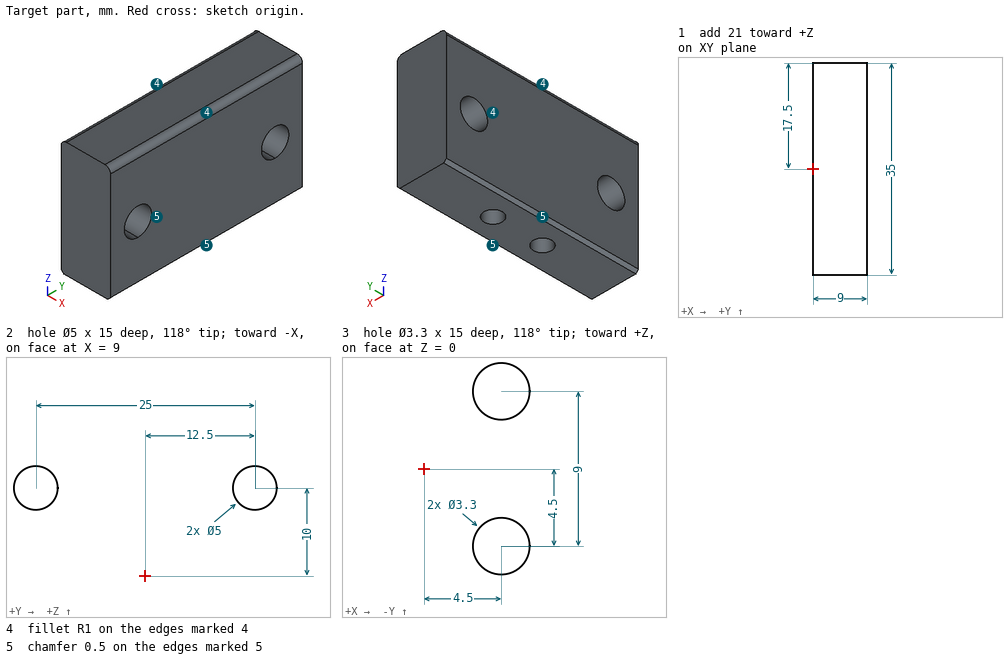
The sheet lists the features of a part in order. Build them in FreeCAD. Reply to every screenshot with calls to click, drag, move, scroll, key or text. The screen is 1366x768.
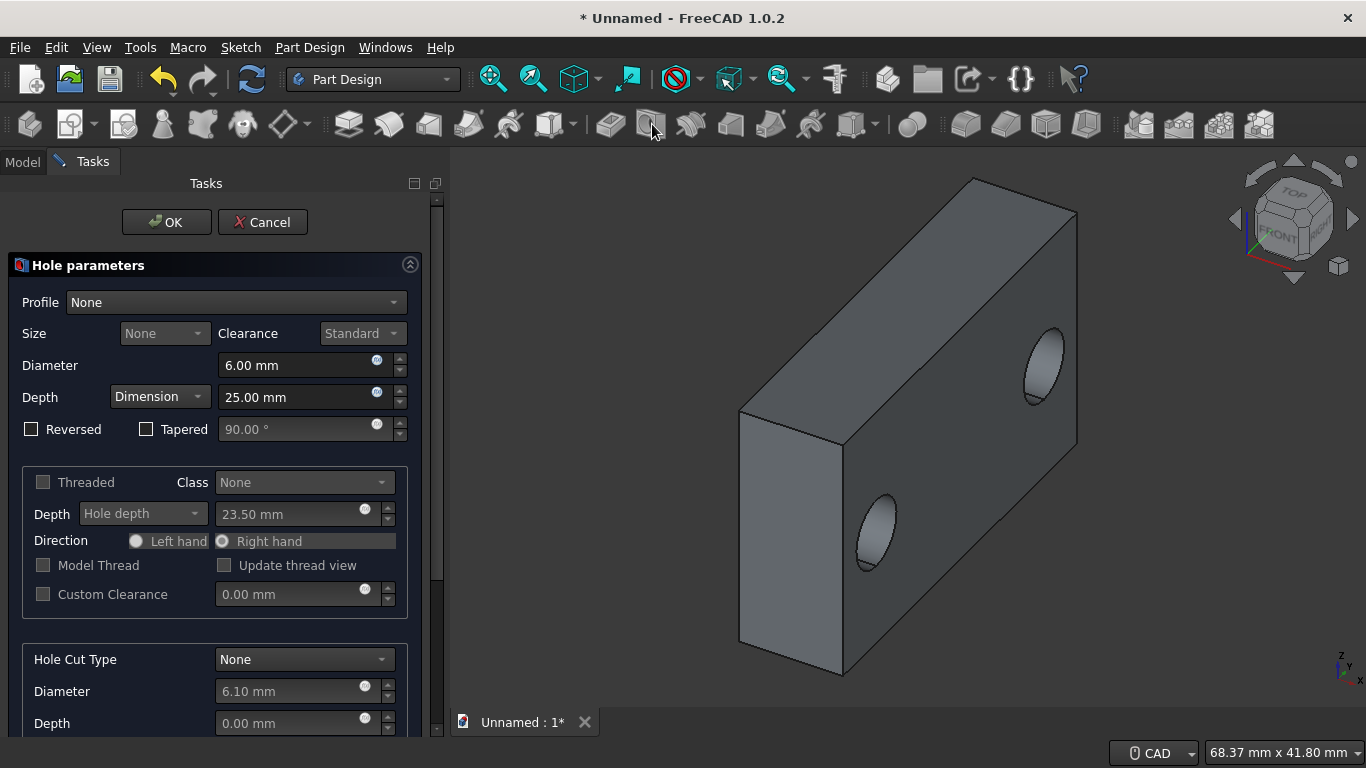
triple_click(305, 365)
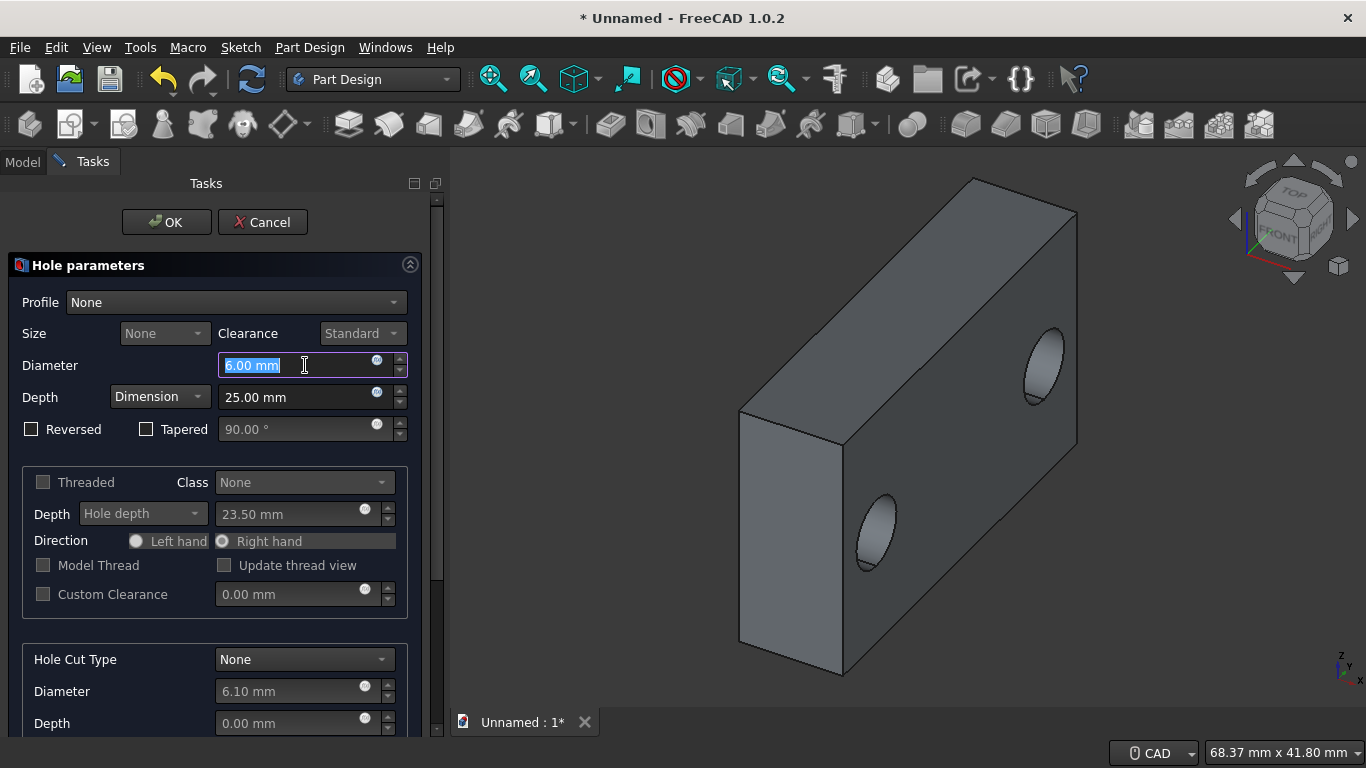
text(5)
key(Tab)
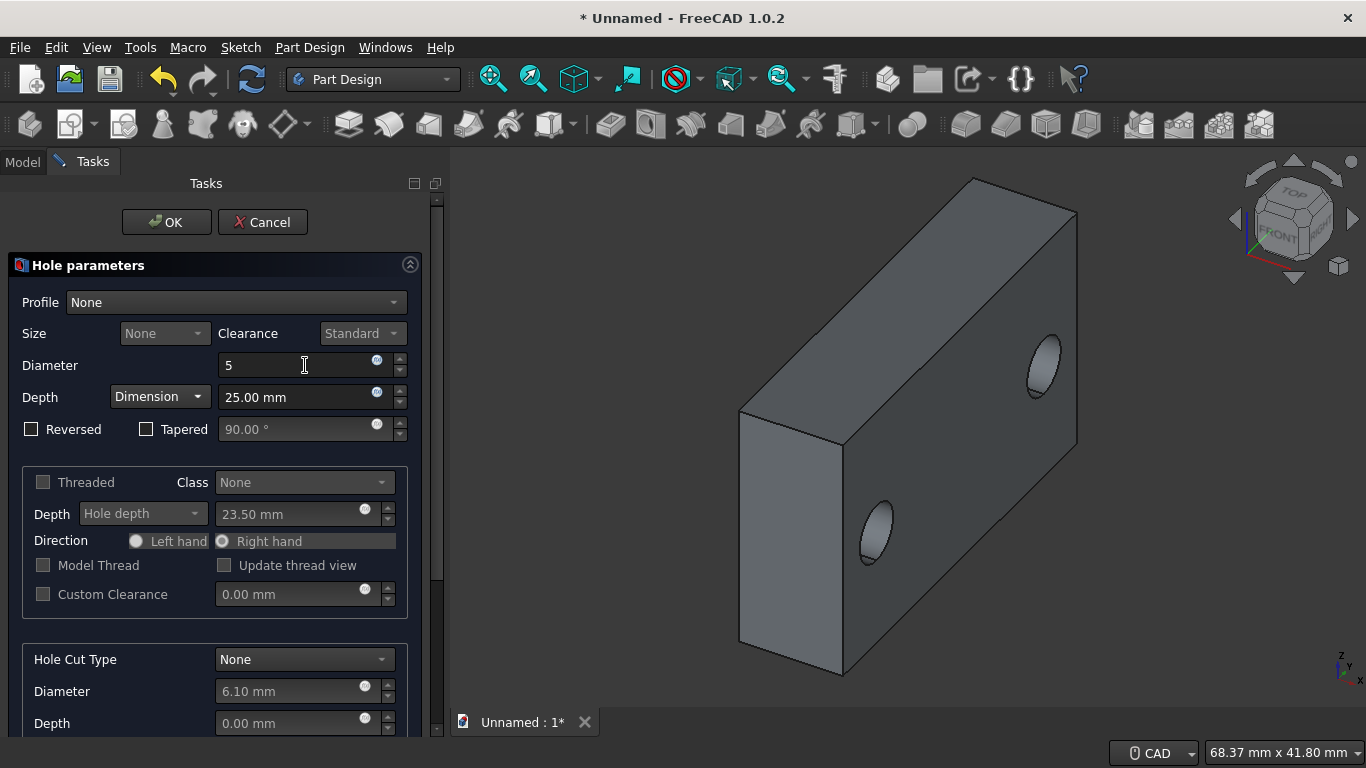
triple_click(305, 397)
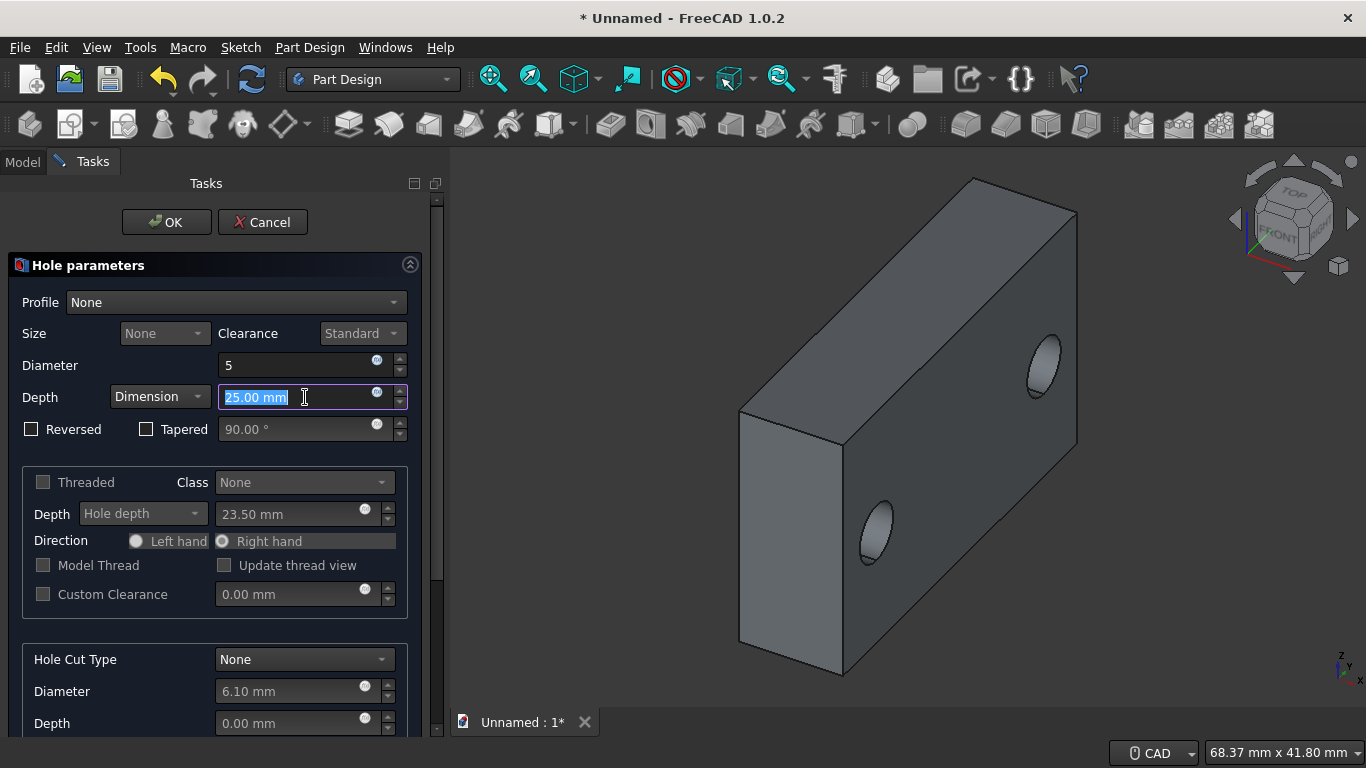
text(15)
key(Tab)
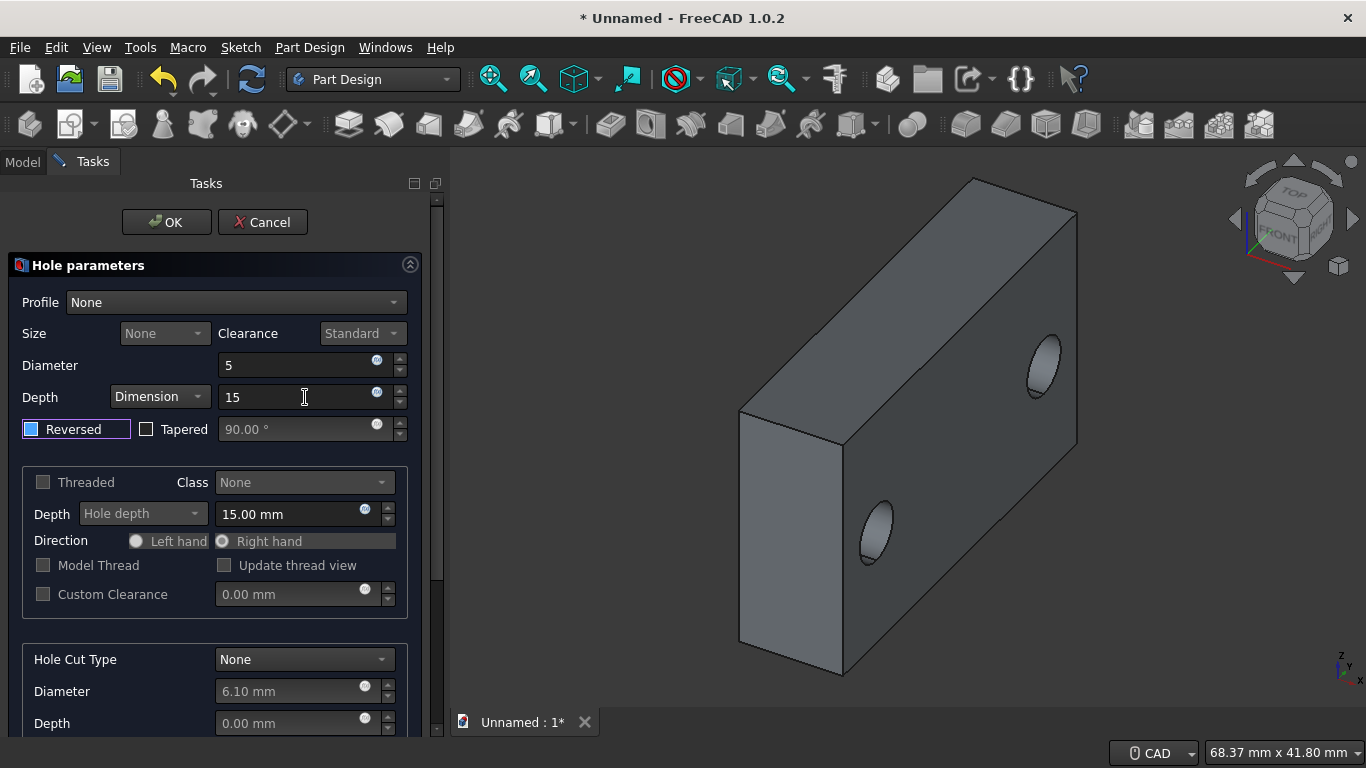
click(167, 222)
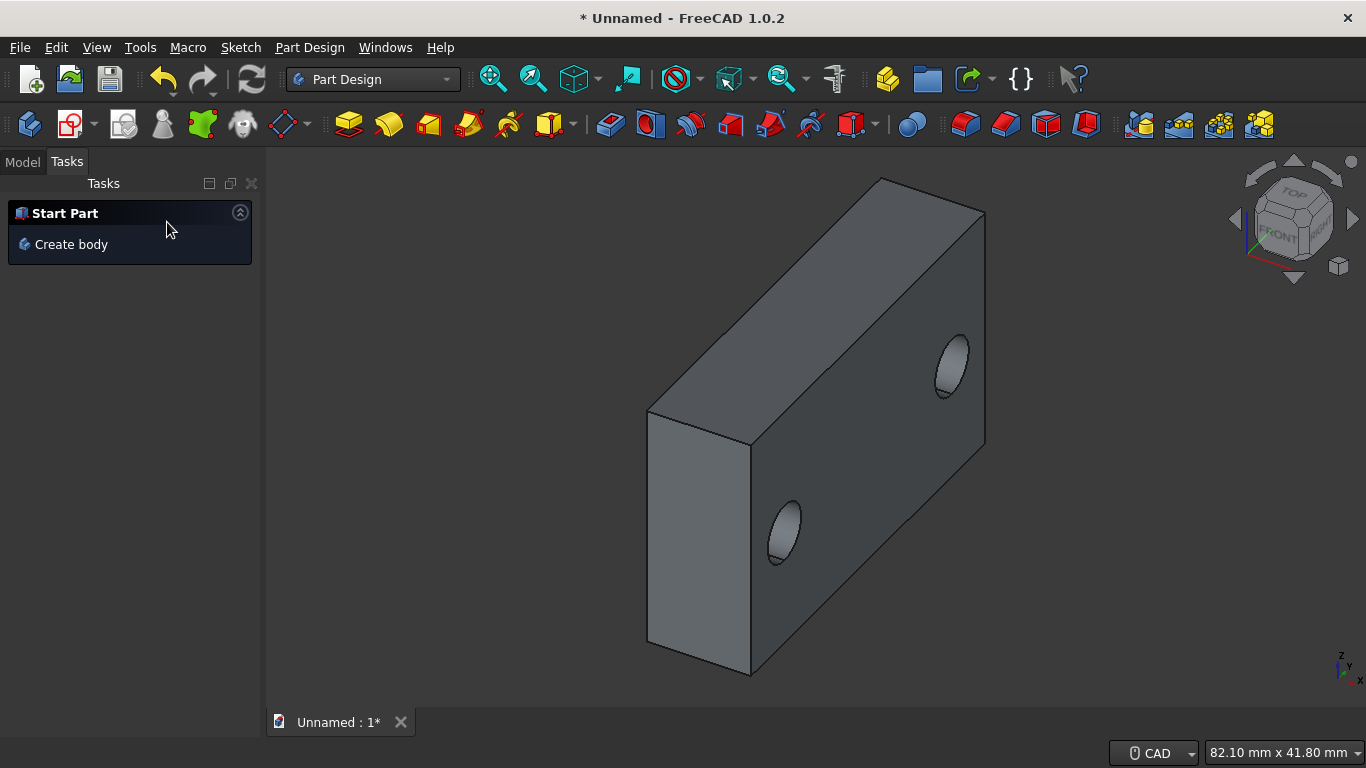
key(5)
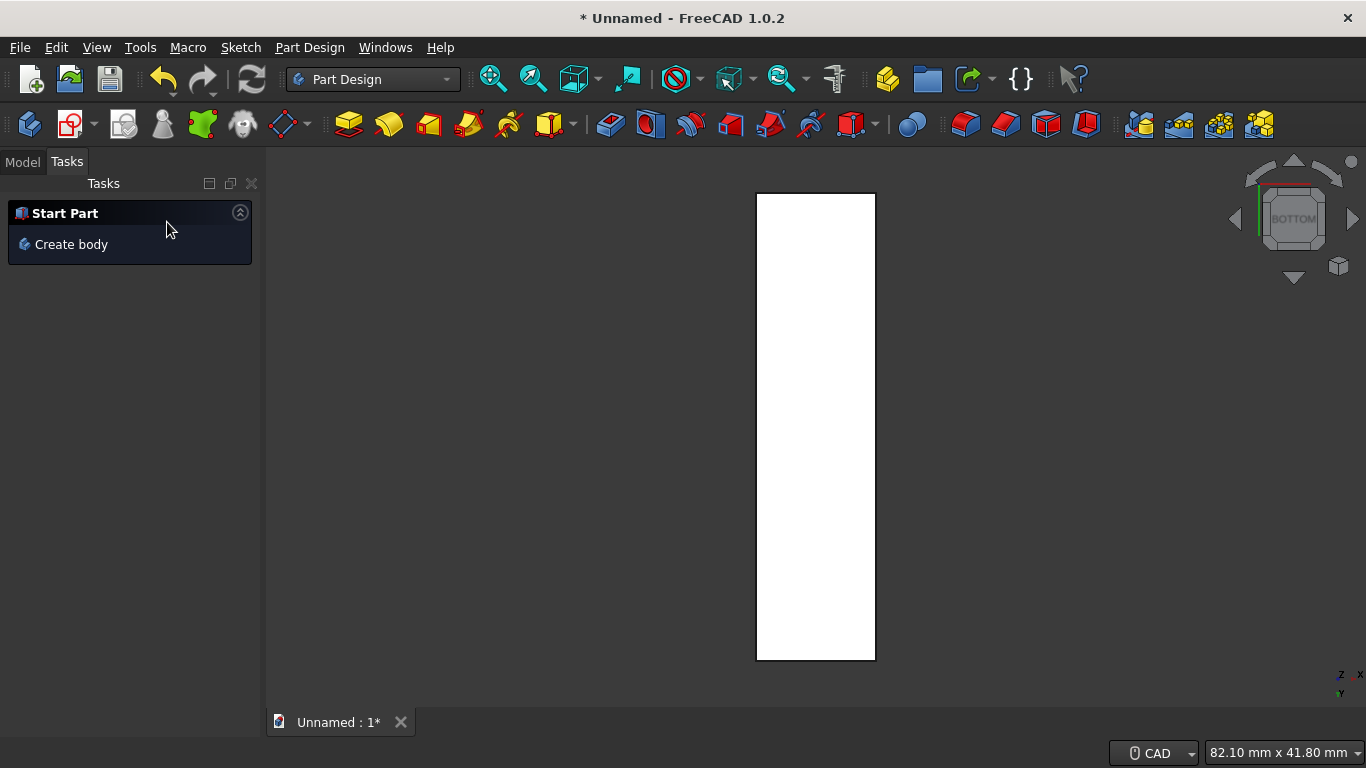
click(816, 560)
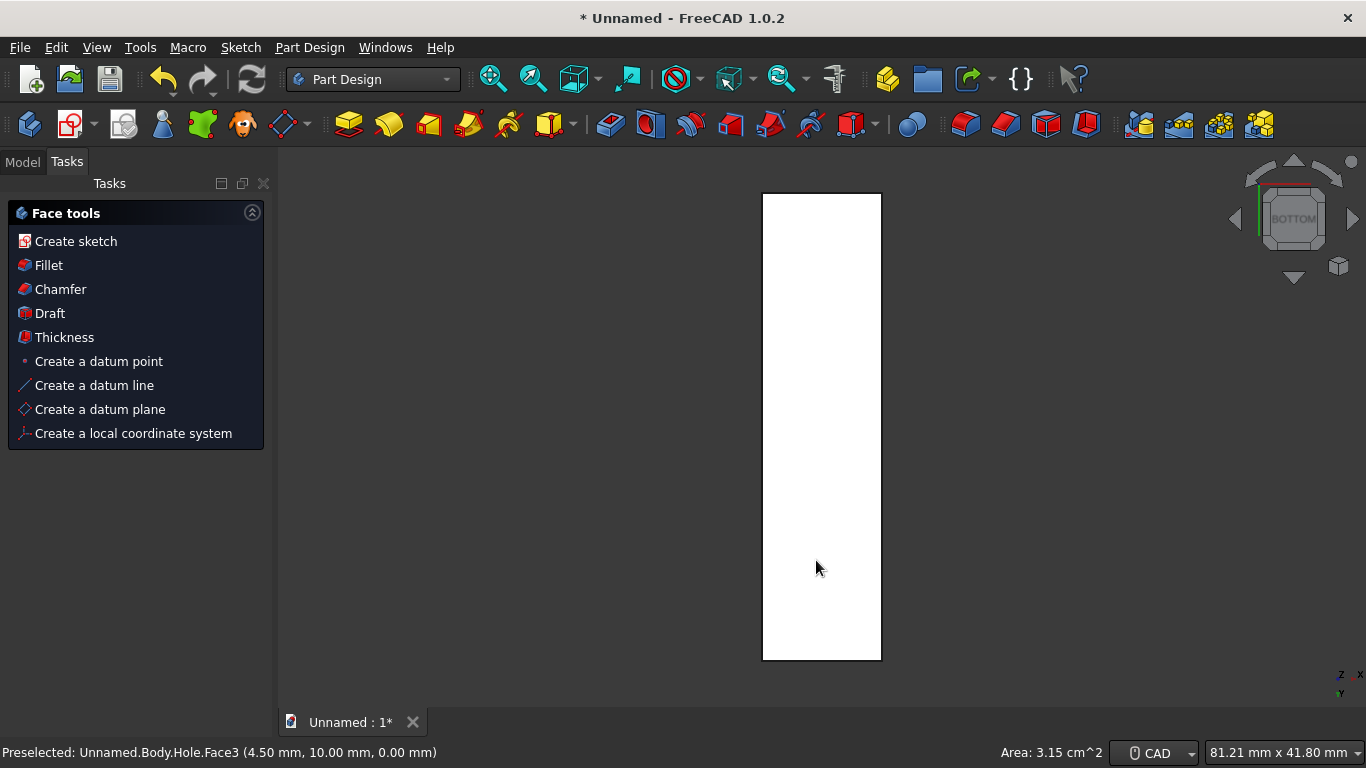
click(70, 124)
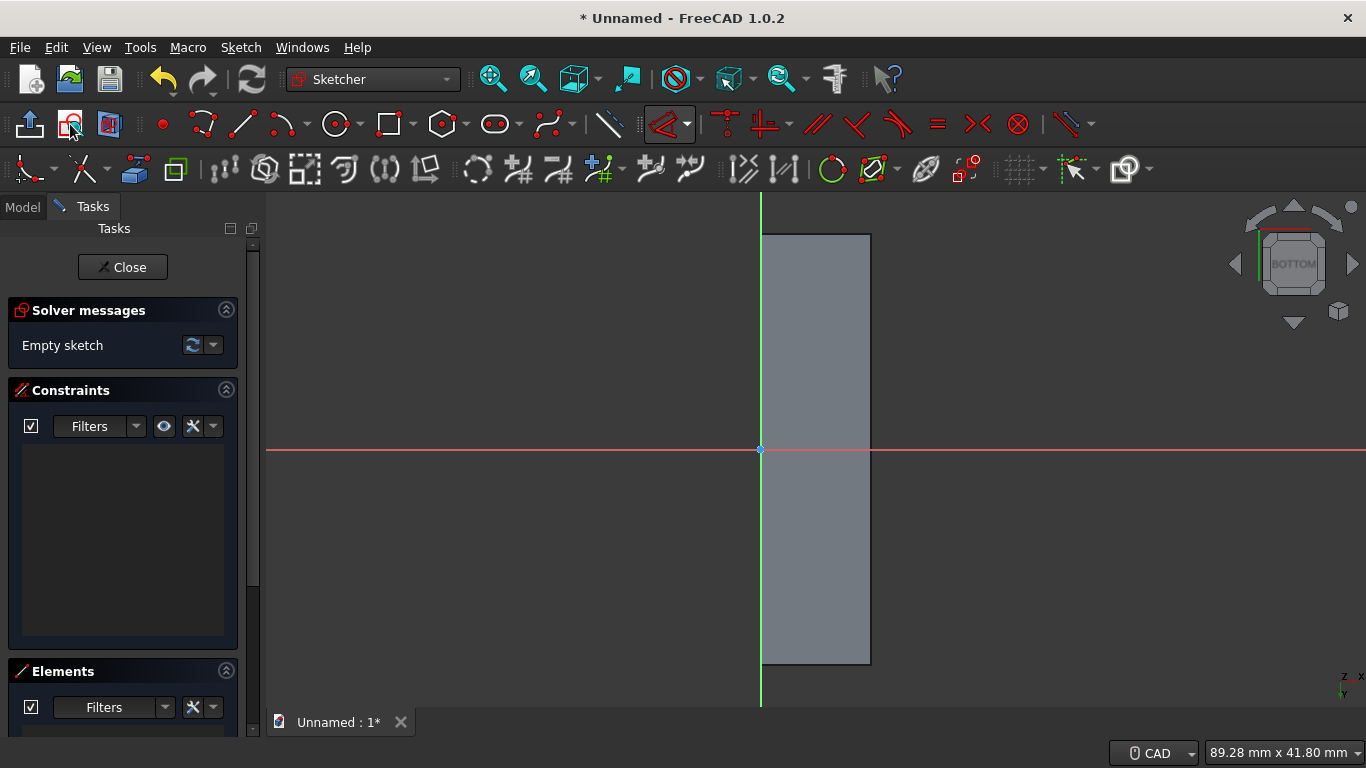
scroll(840, 450, up, 4)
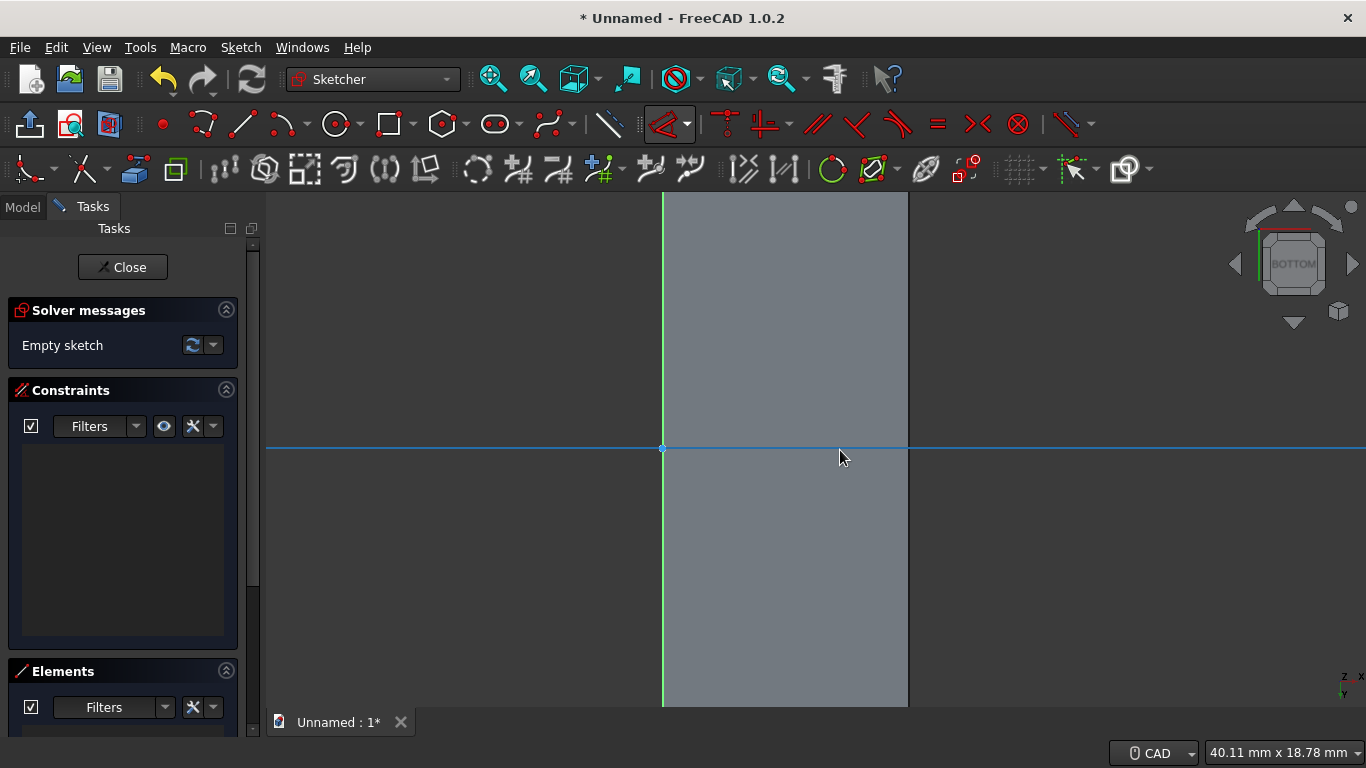
key(g)
key(c)